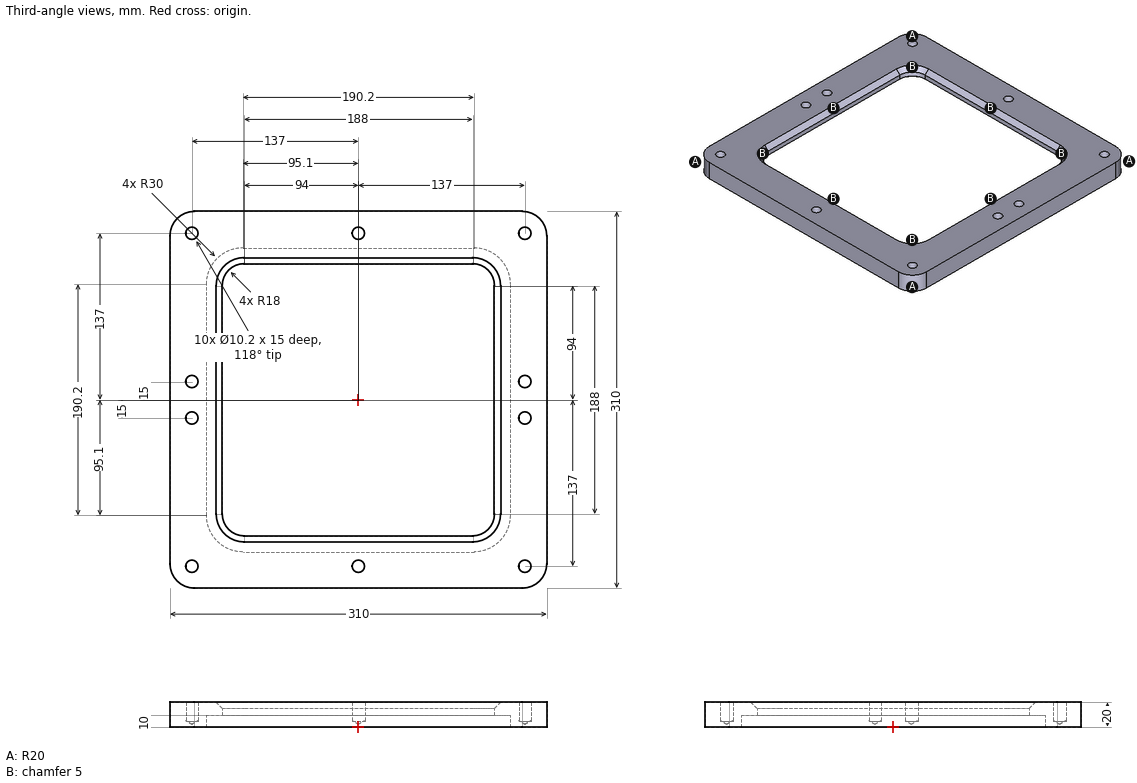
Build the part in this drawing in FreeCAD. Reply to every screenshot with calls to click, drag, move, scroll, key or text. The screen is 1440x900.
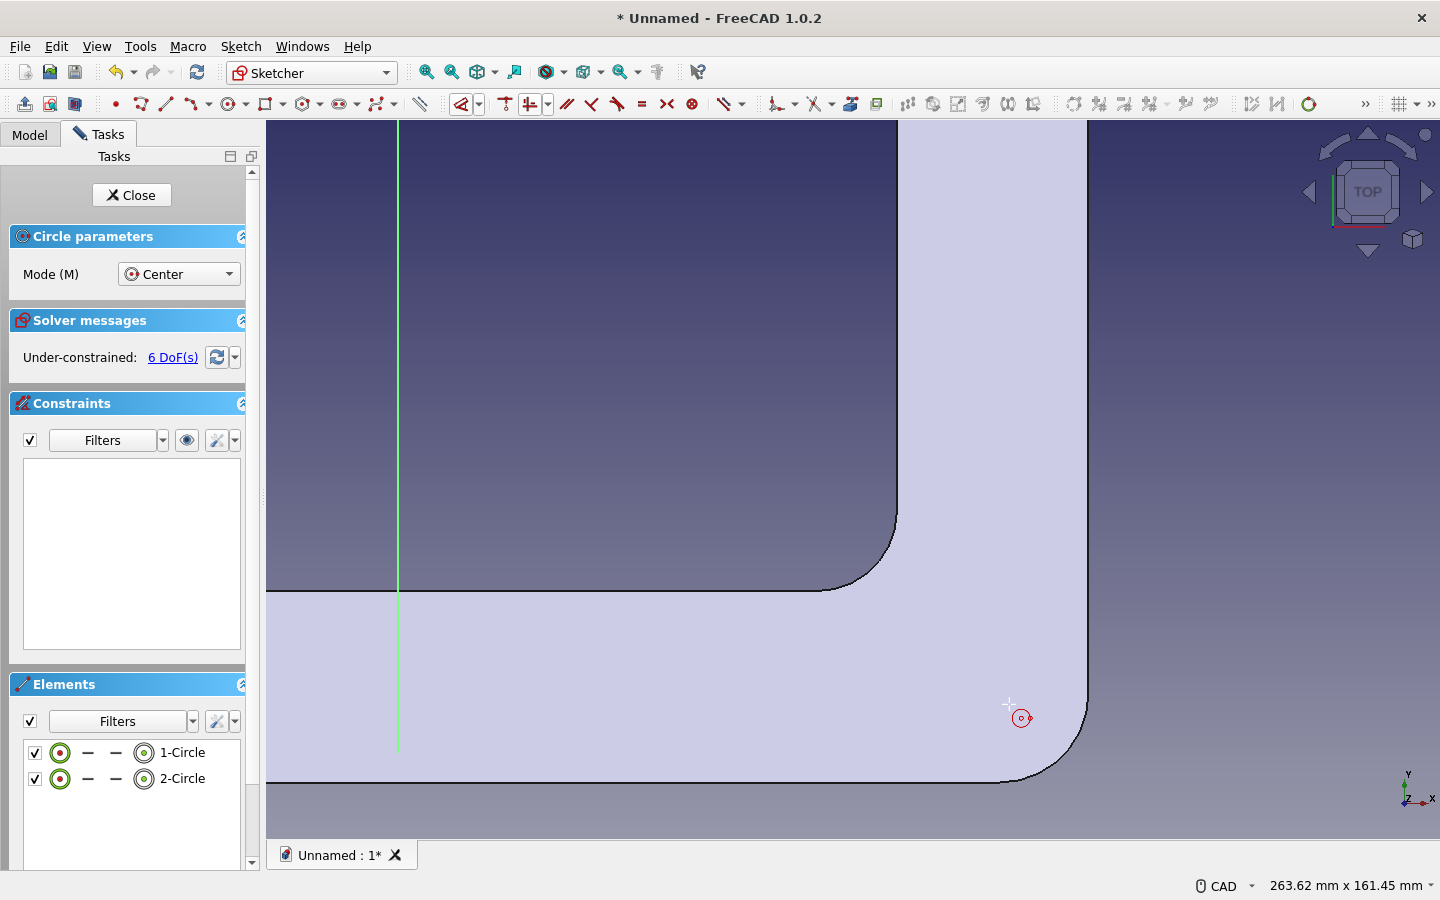
click(1008, 702)
click(1024, 686)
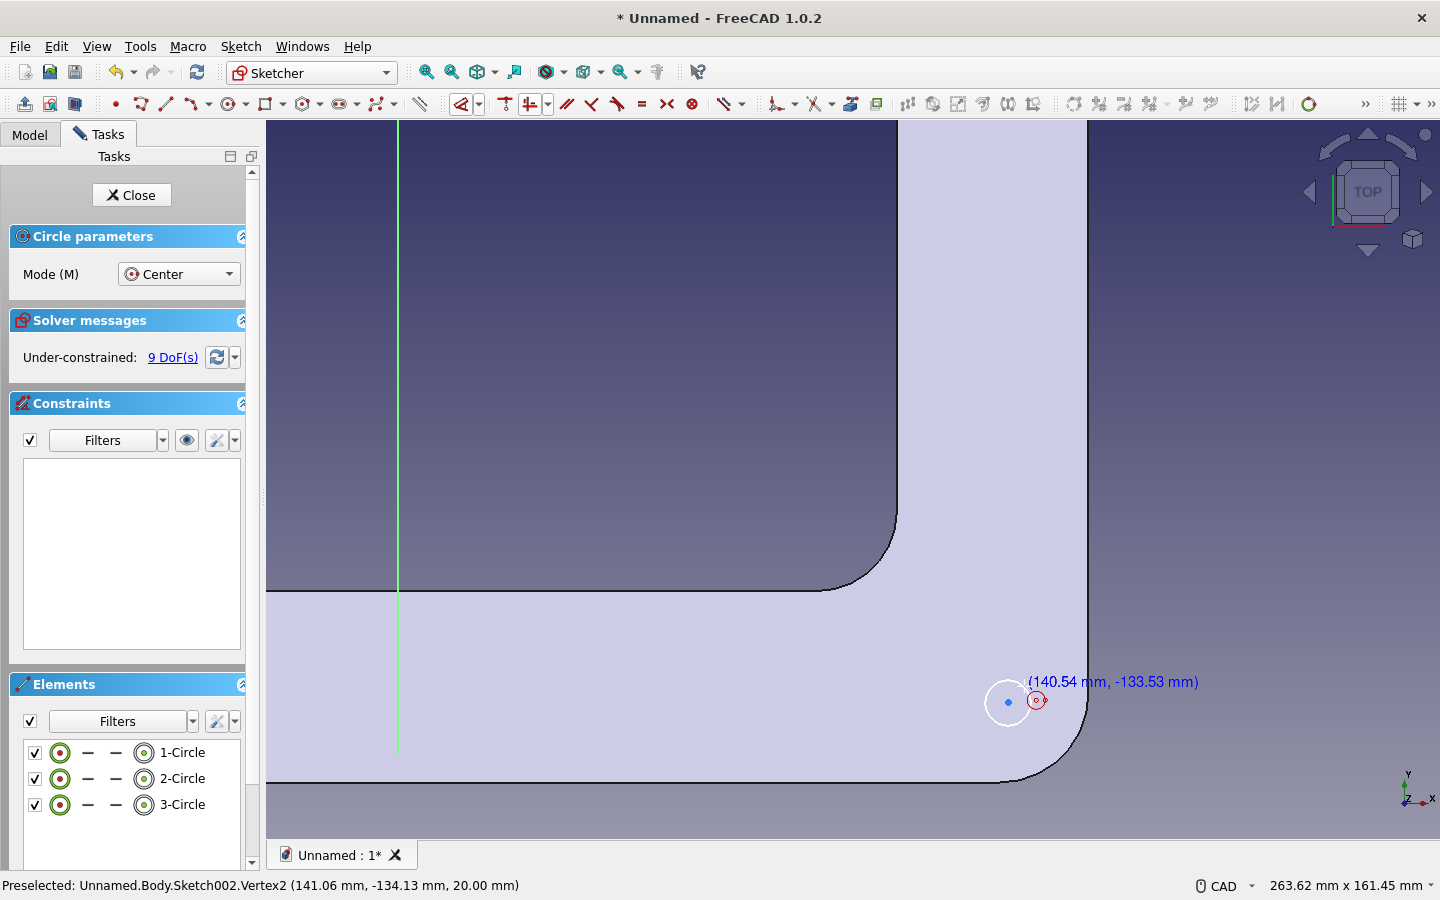
scroll(1009, 705, down, 5)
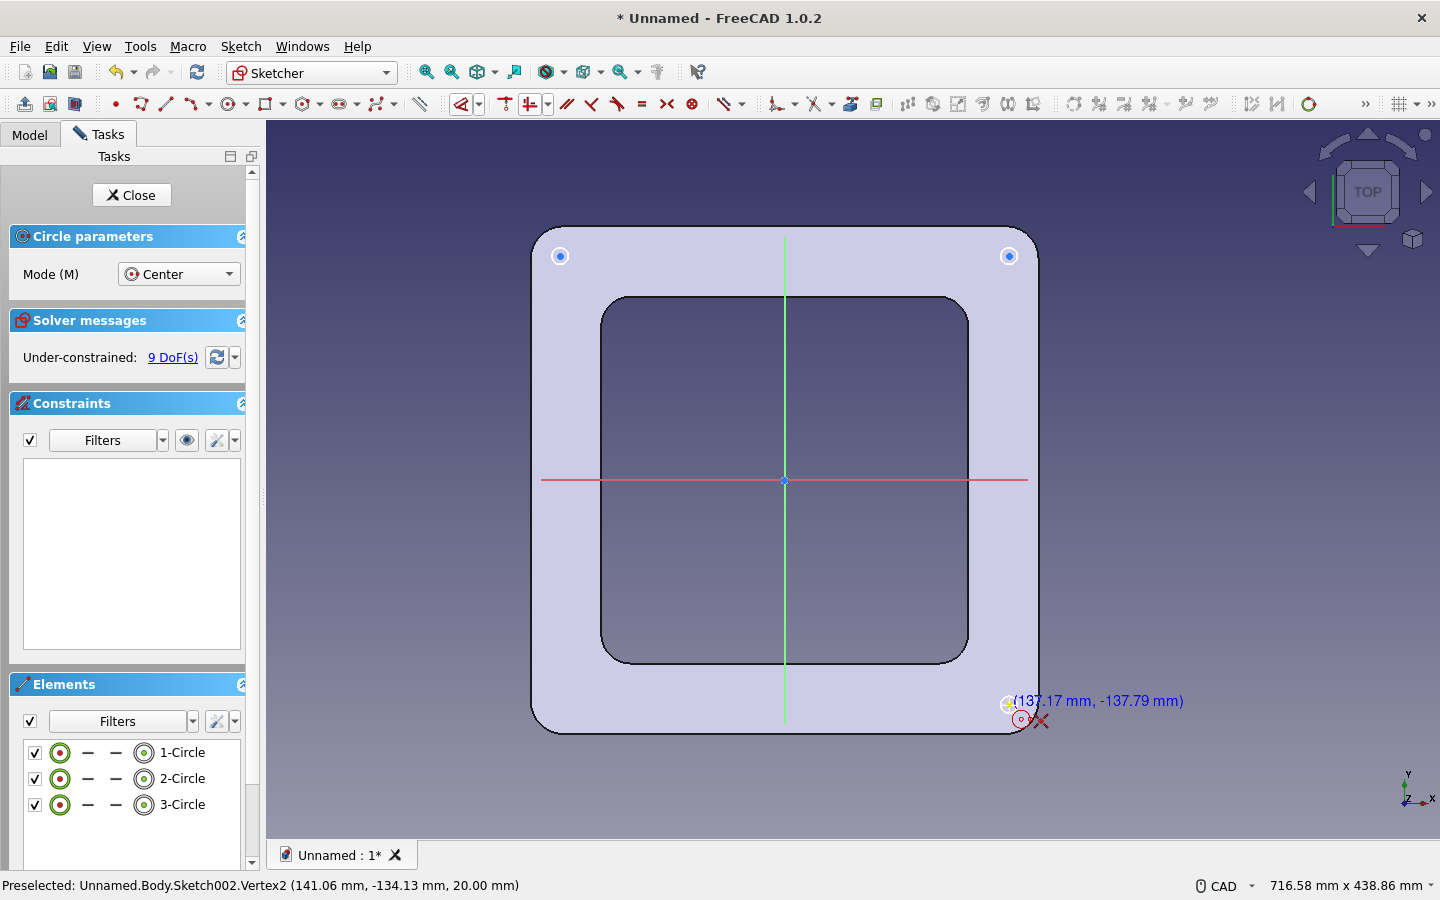
scroll(560, 705, up, 5)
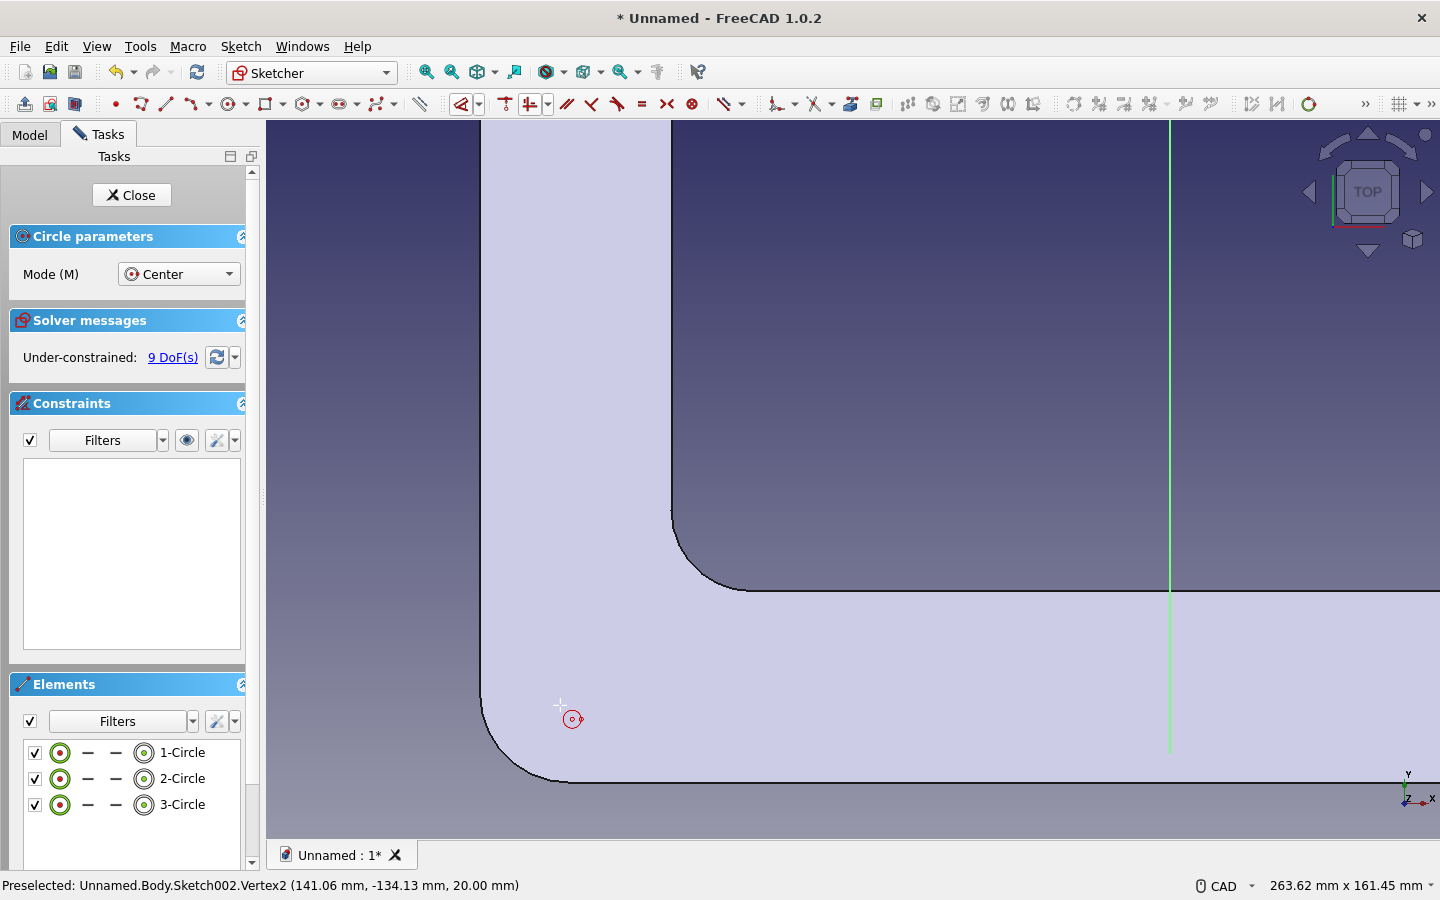
click(560, 702)
click(576, 686)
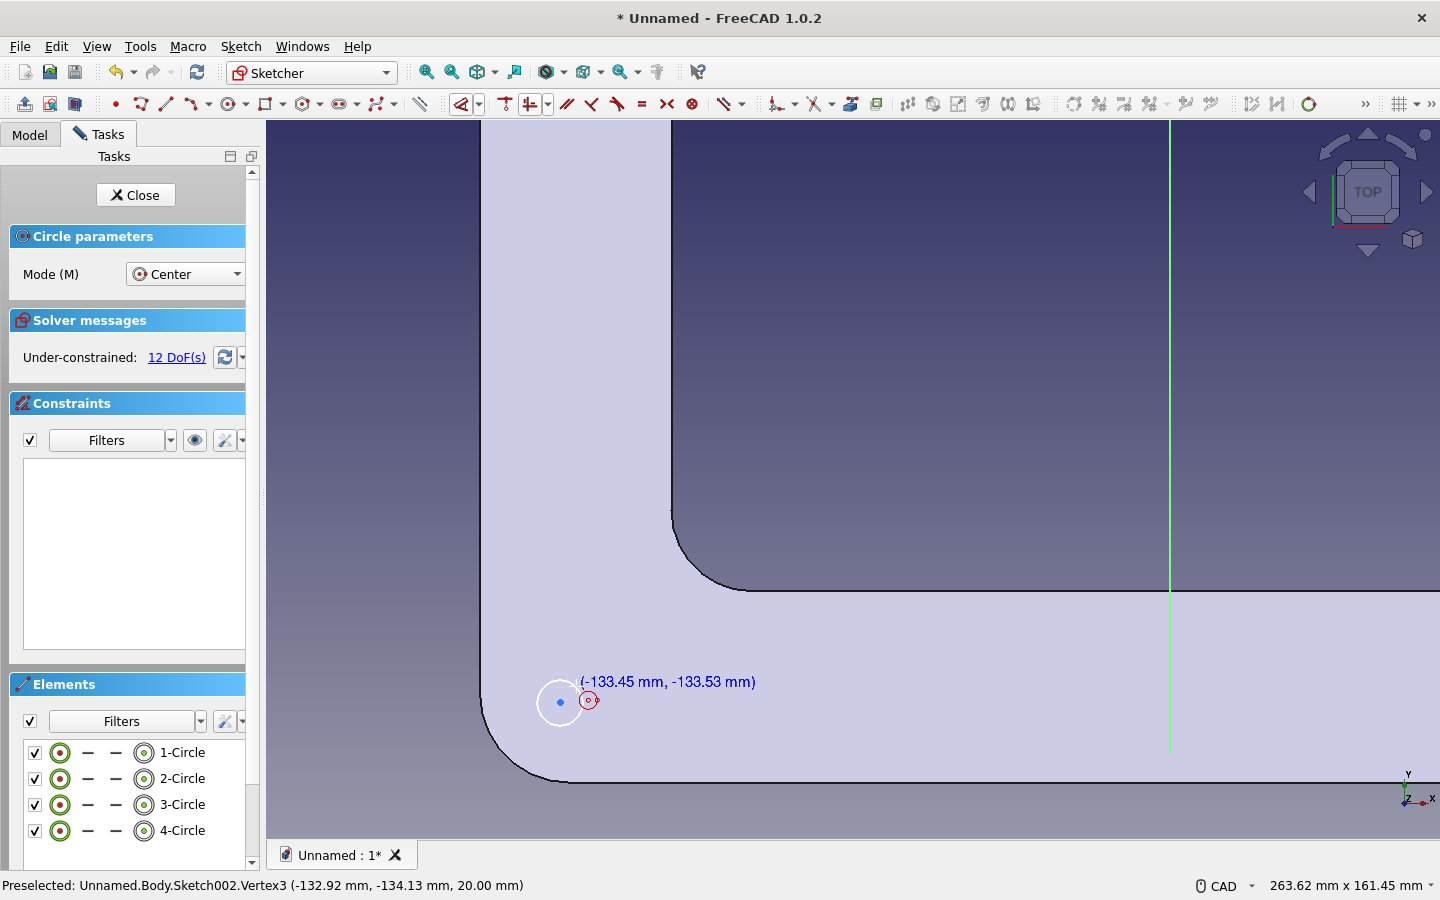
click(1170, 702)
click(1186, 686)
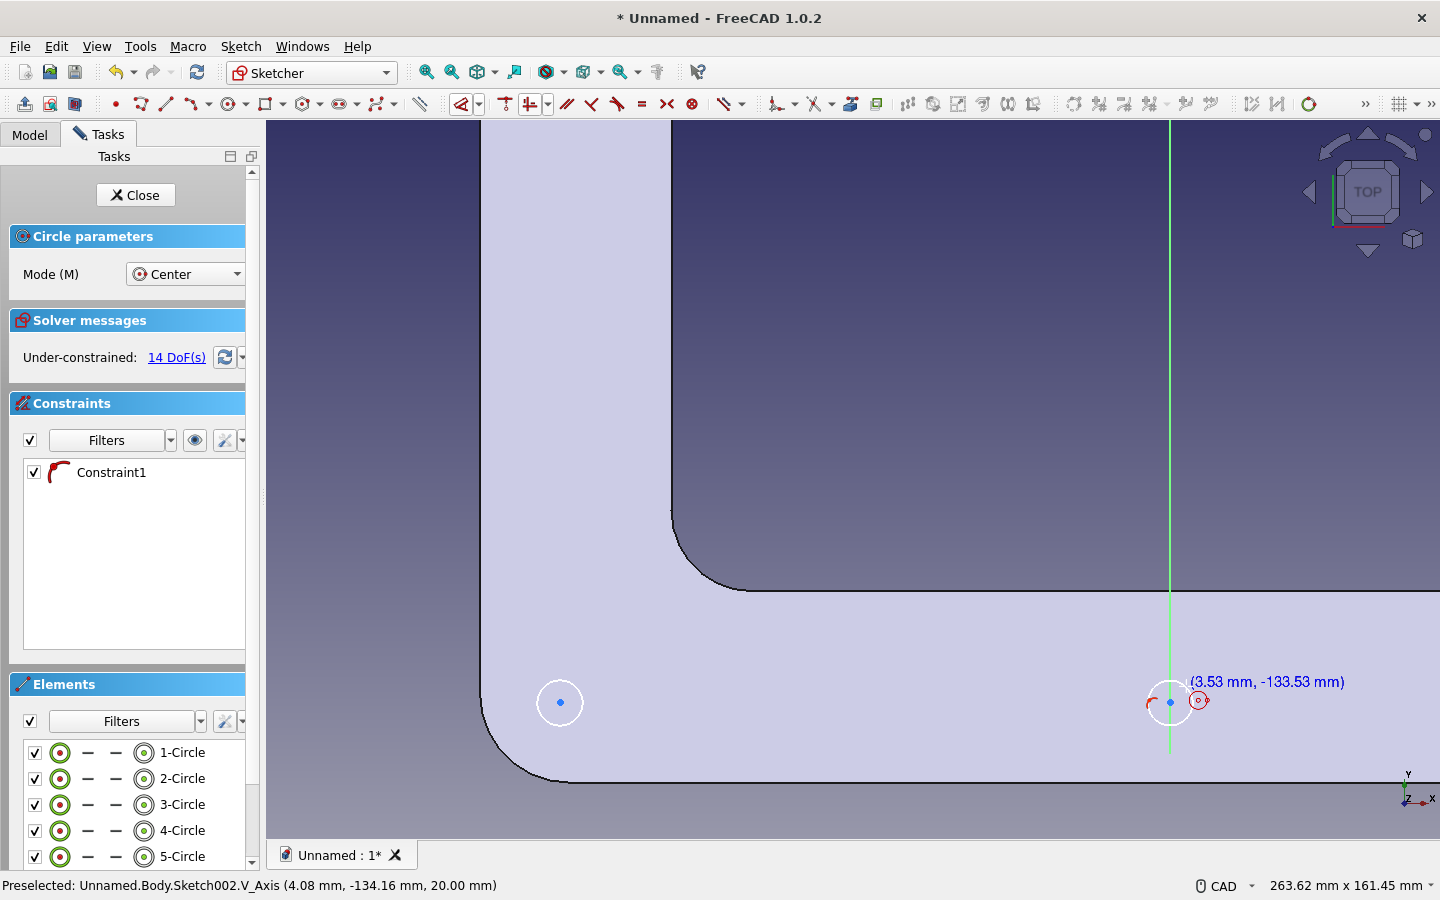
scroll(560, 705, down, 5)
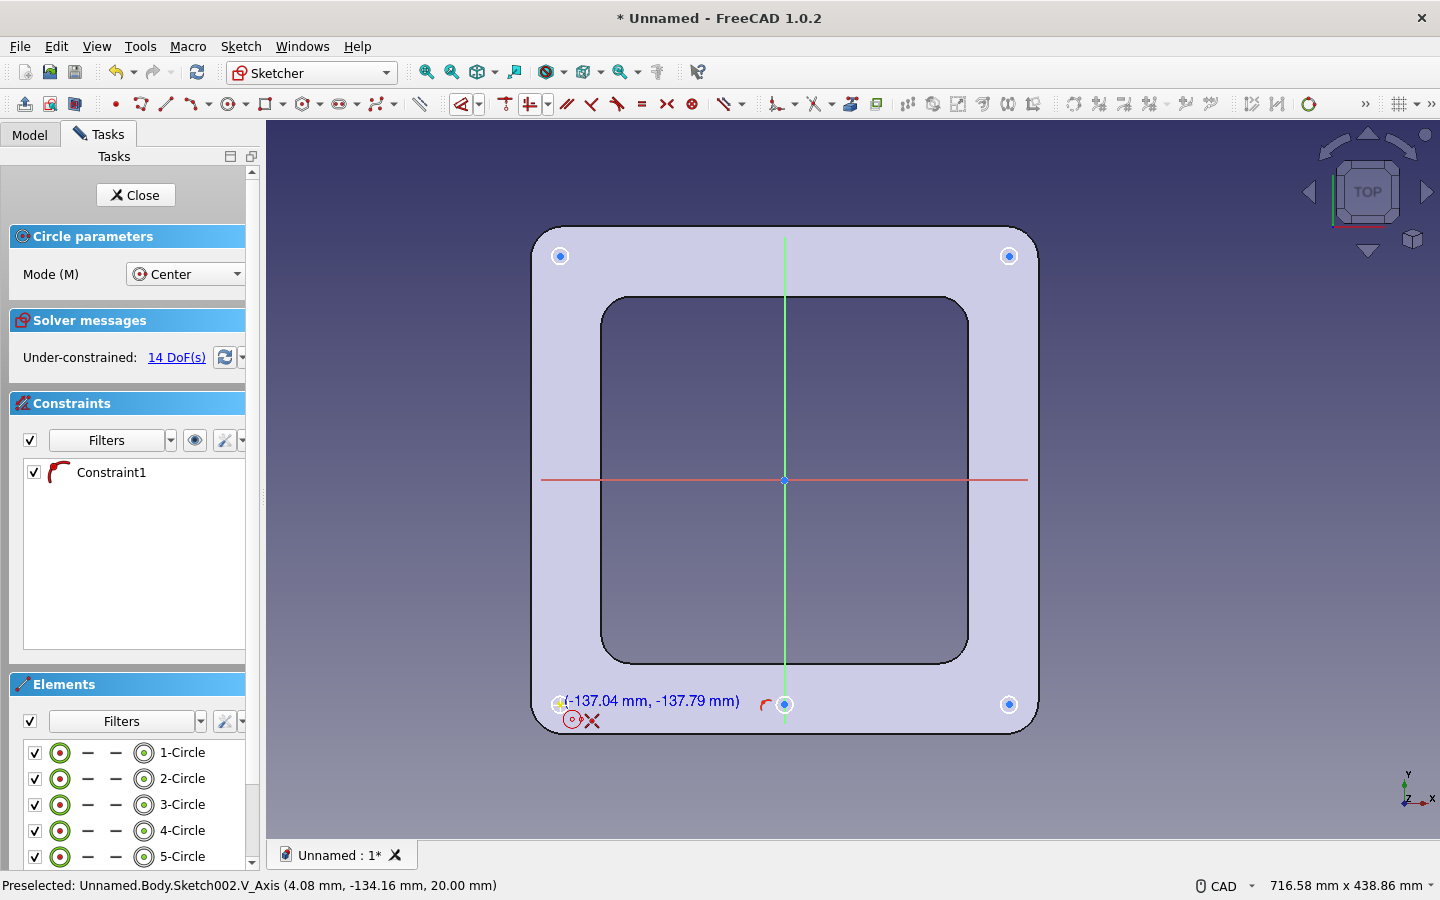
scroll(785, 256, up, 5)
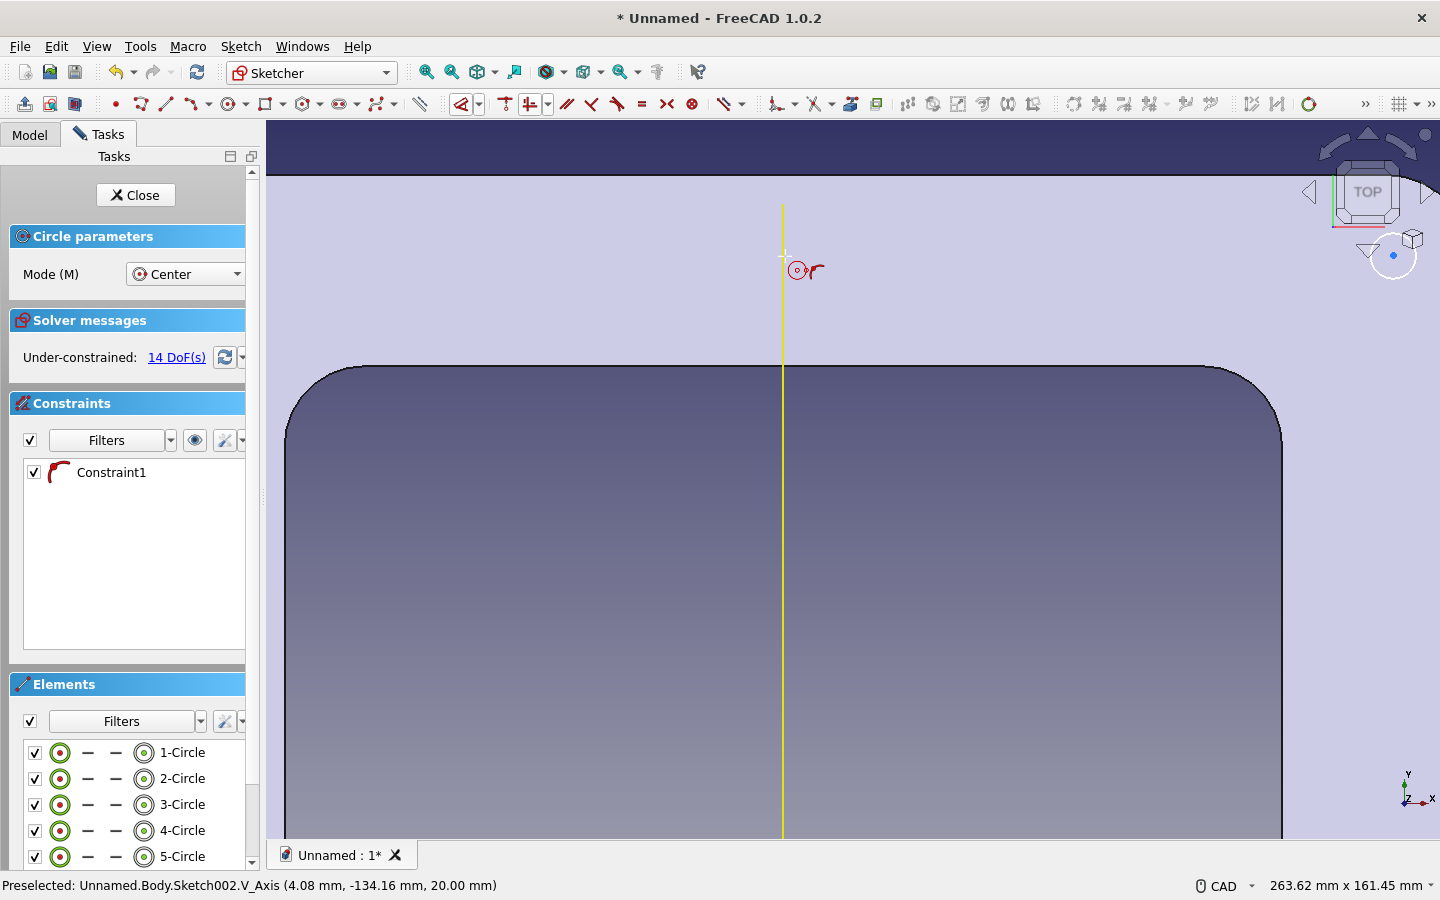
click(783, 255)
click(799, 239)